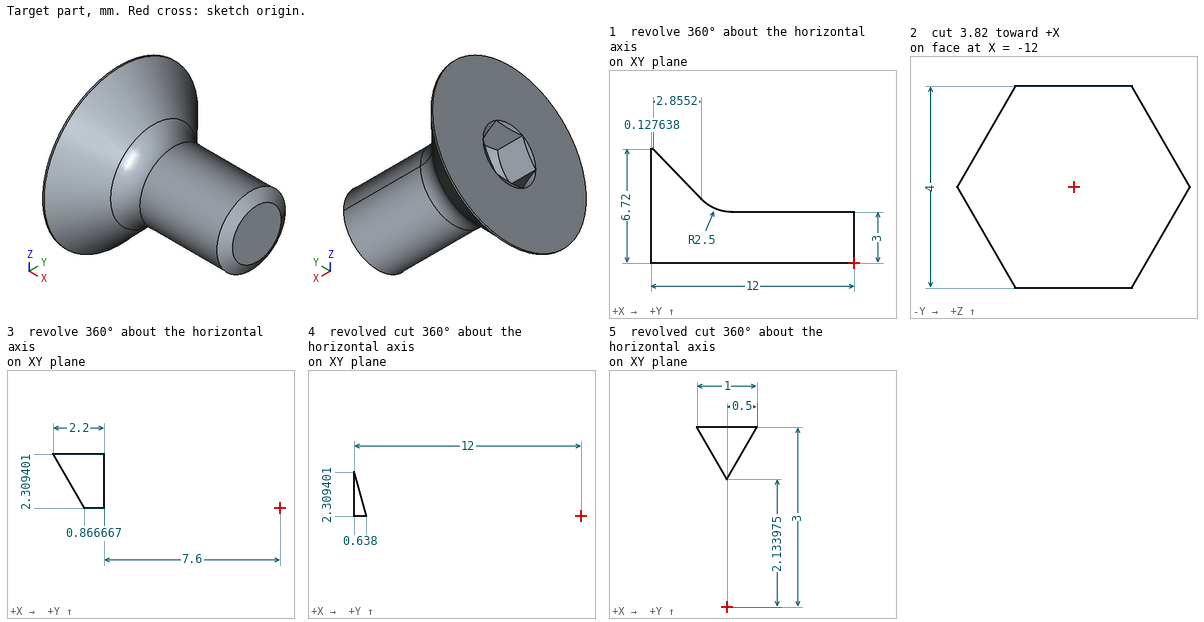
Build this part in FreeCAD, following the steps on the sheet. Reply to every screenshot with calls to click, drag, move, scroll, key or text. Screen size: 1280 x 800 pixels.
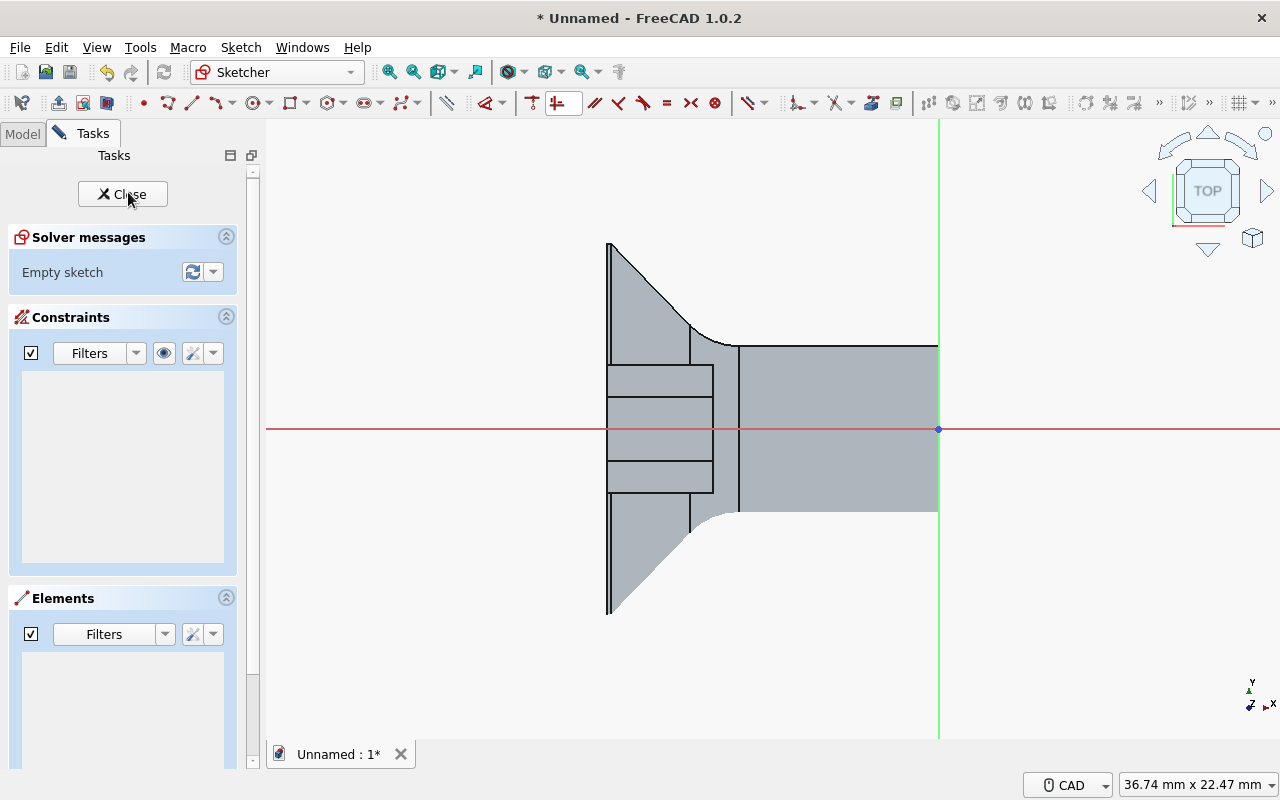
scroll(697, 391, up, 9)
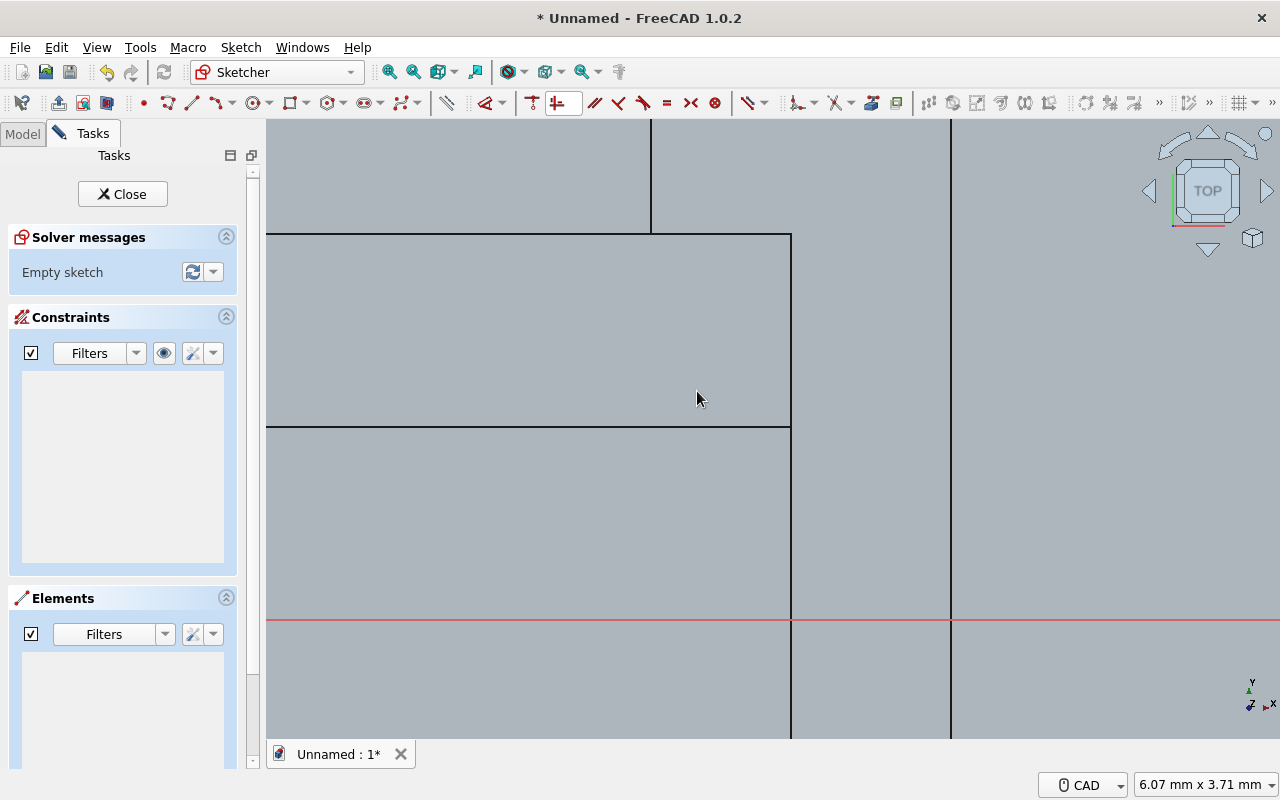
key(g)
key(m)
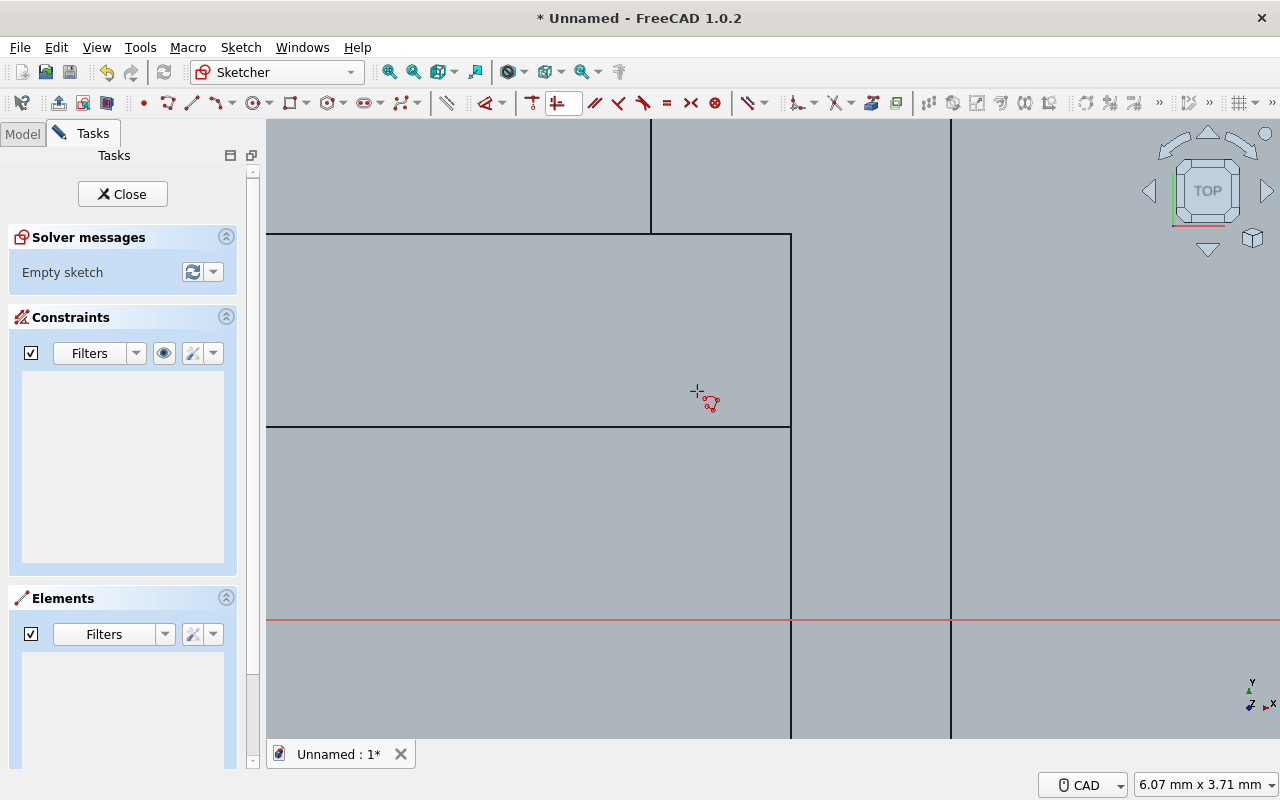
click(888, 620)
click(888, 234)
click(520, 234)
click(743, 611)
click(888, 620)
key(Escape)
key(Escape)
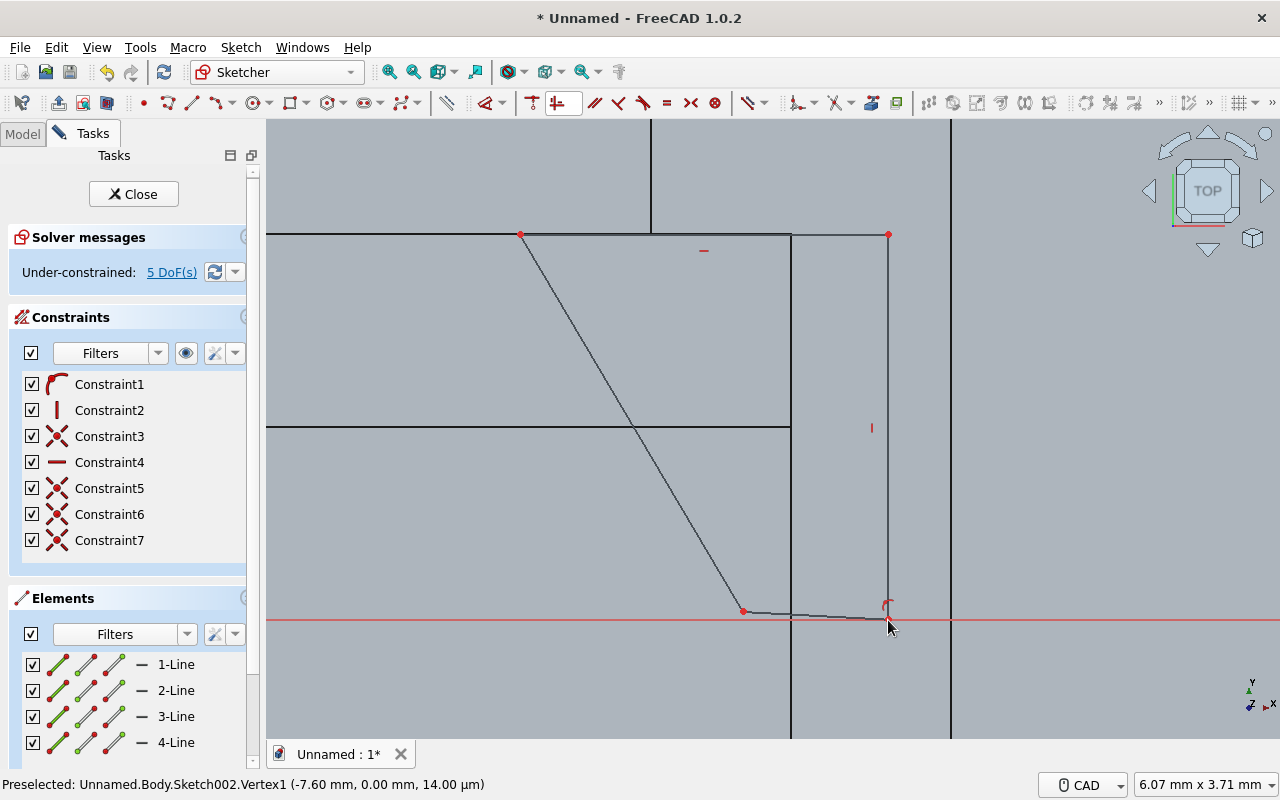
click(845, 617)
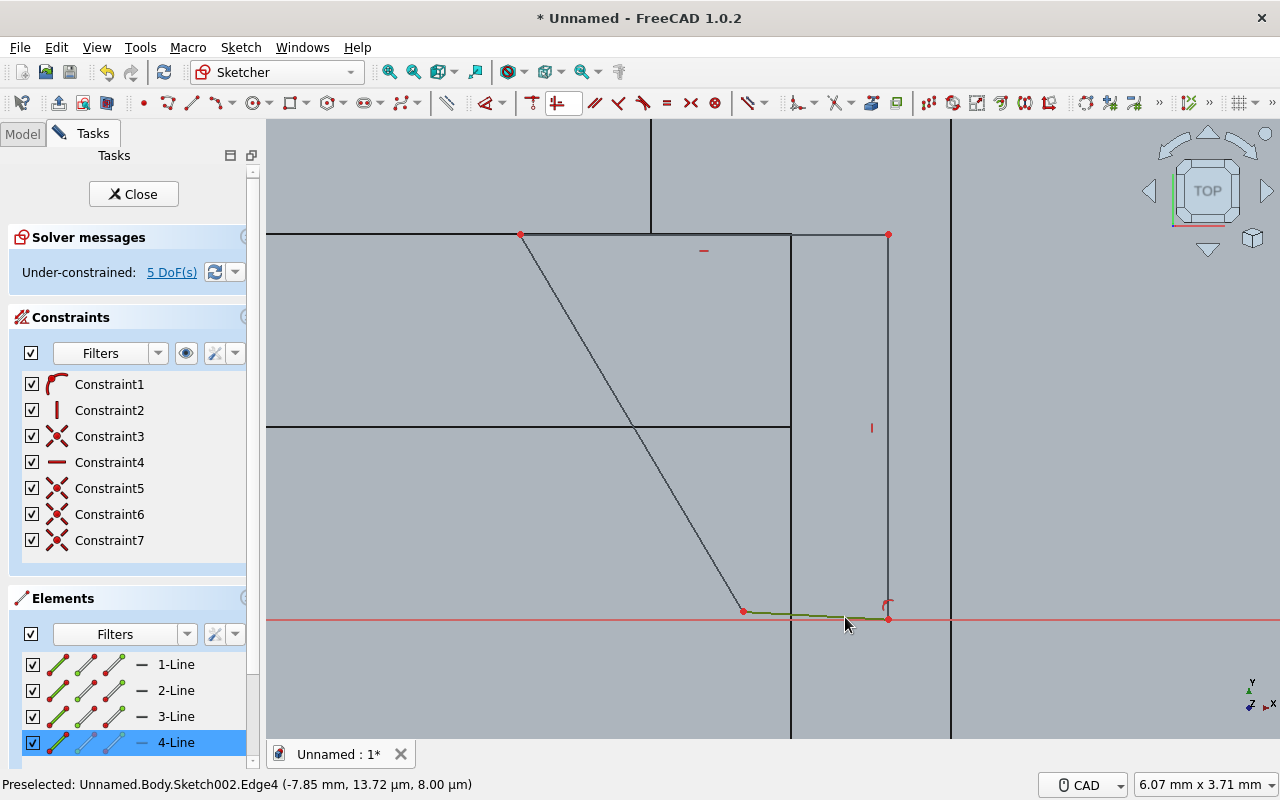
click(576, 104)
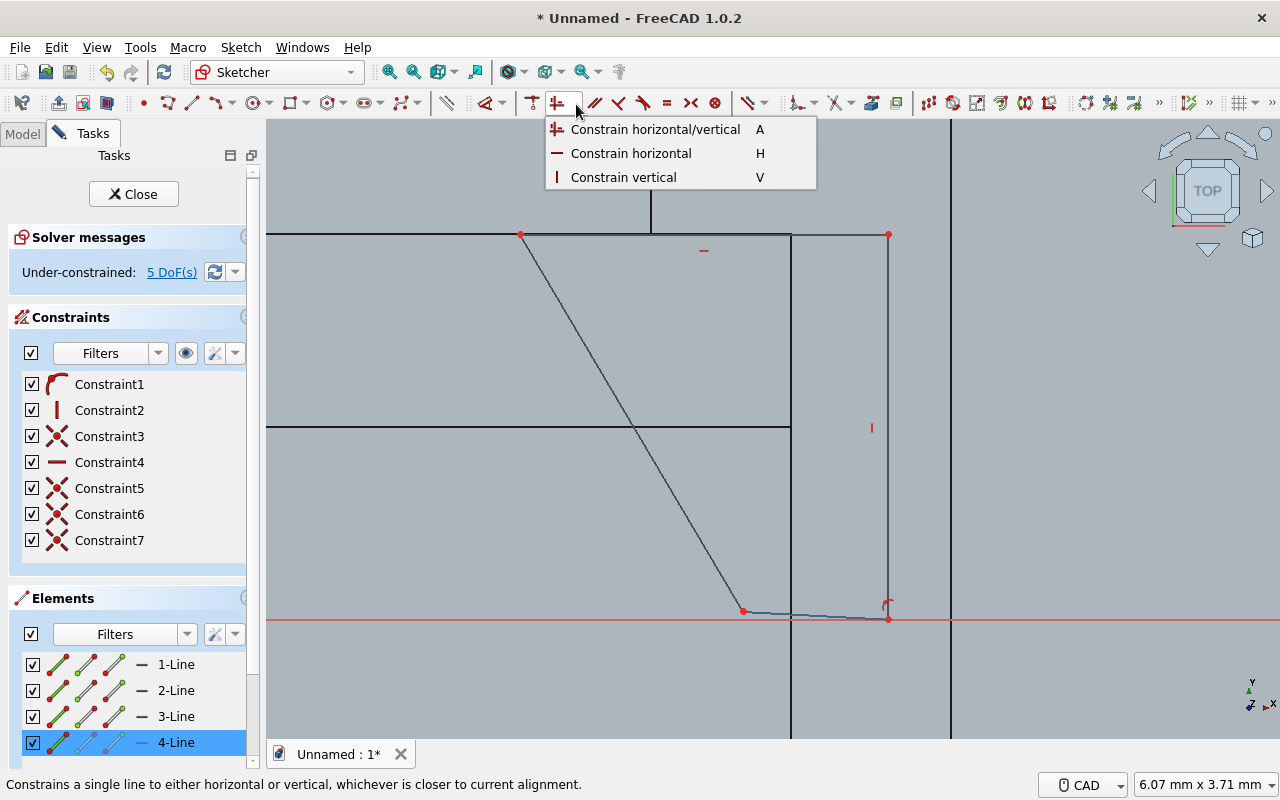
click(681, 153)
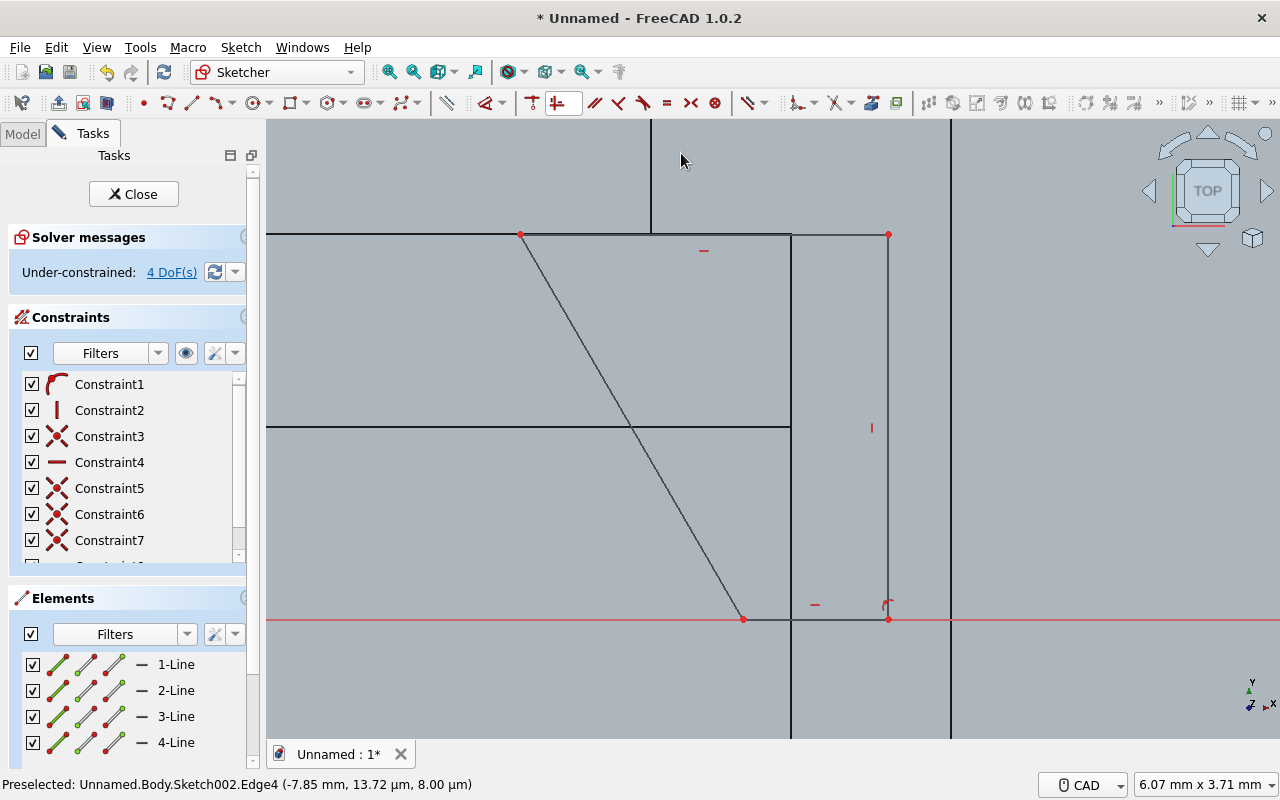
key(d)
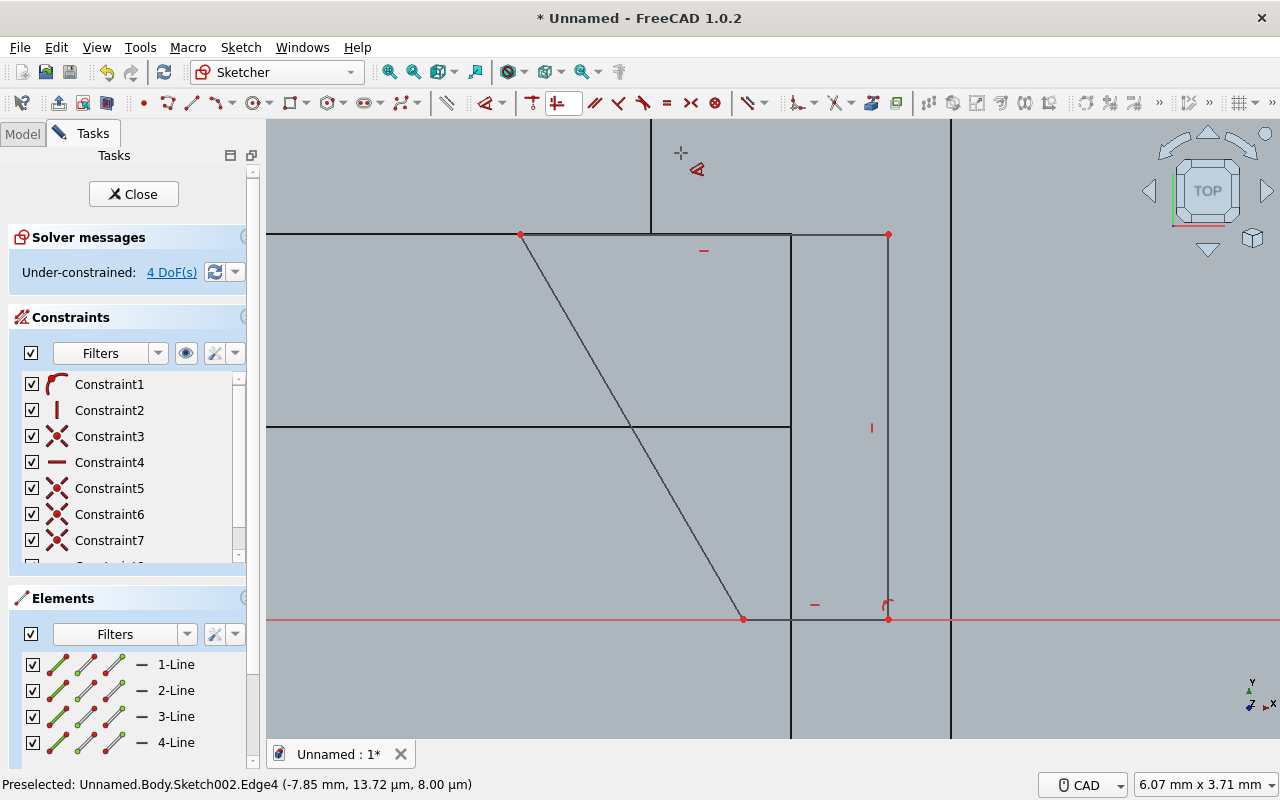
click(778, 235)
click(704, 201)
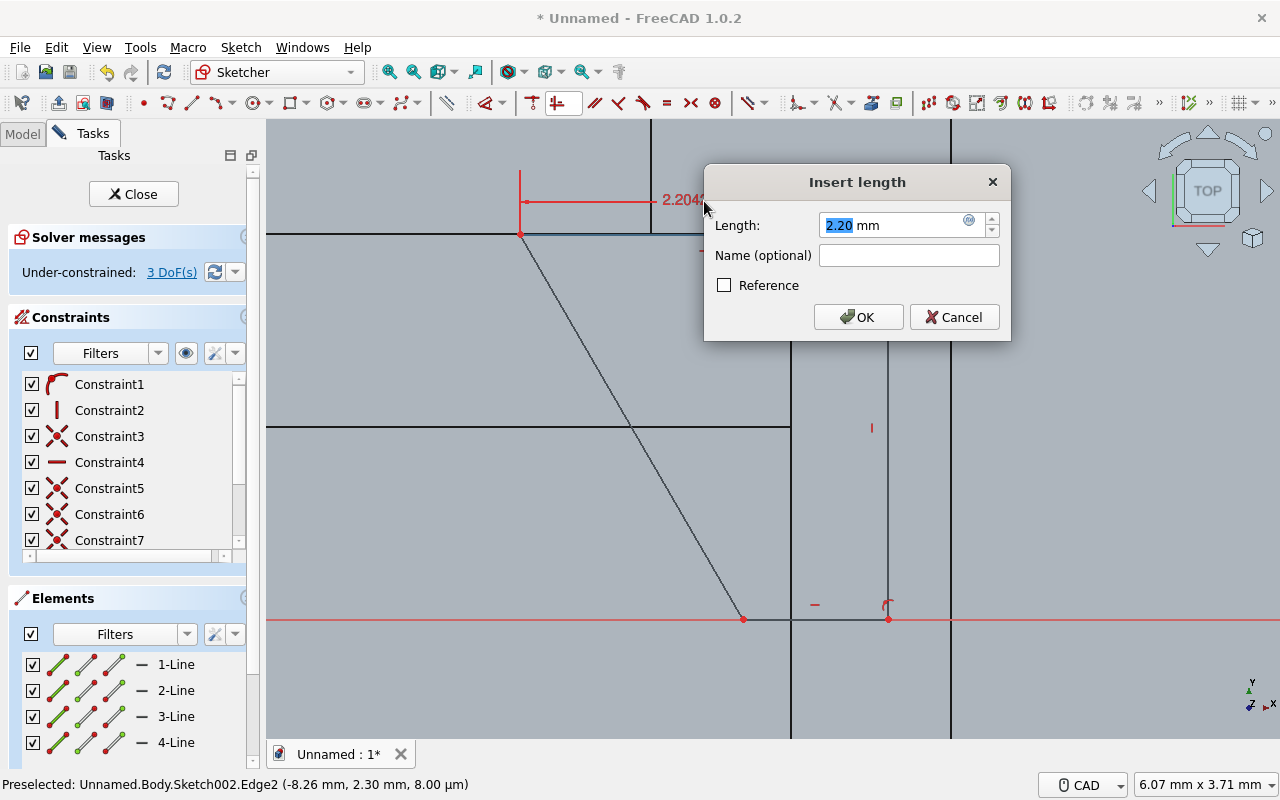
text(2.2)
key(Return)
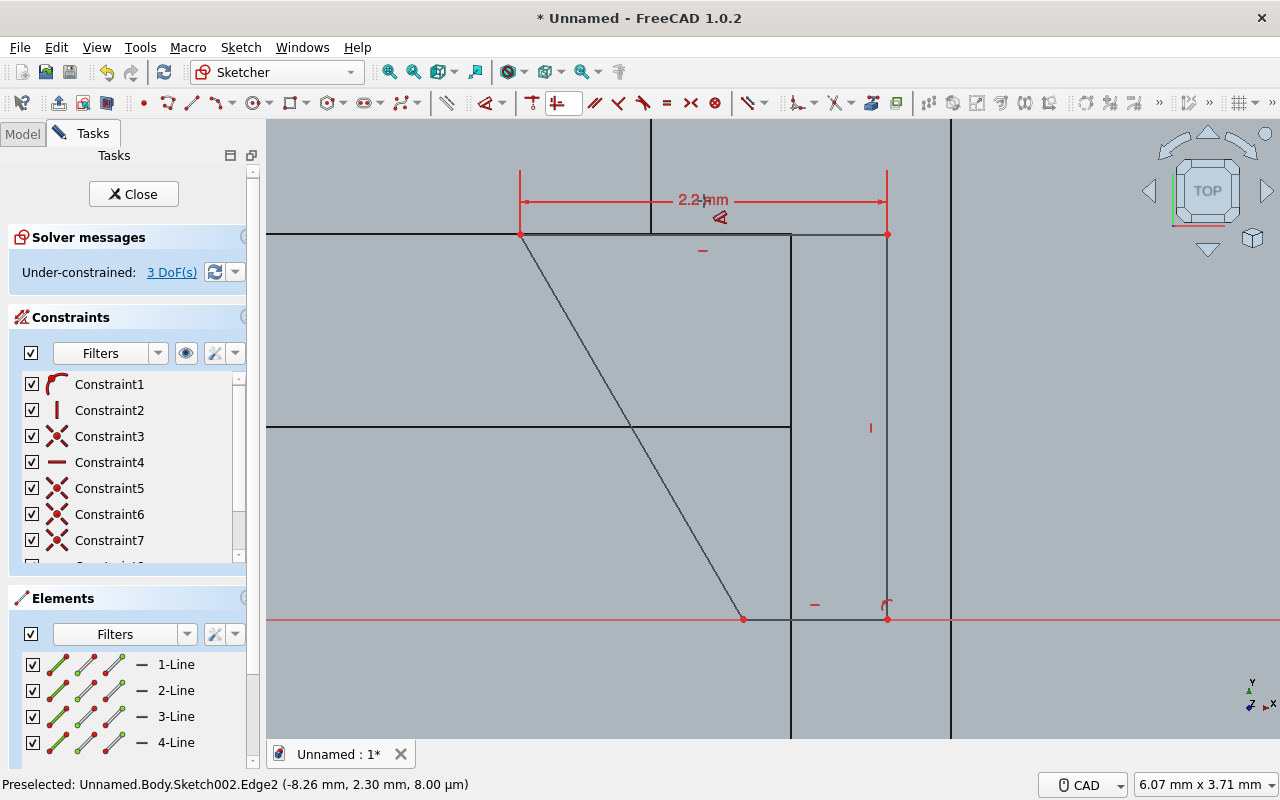
click(887, 620)
click(1001, 654)